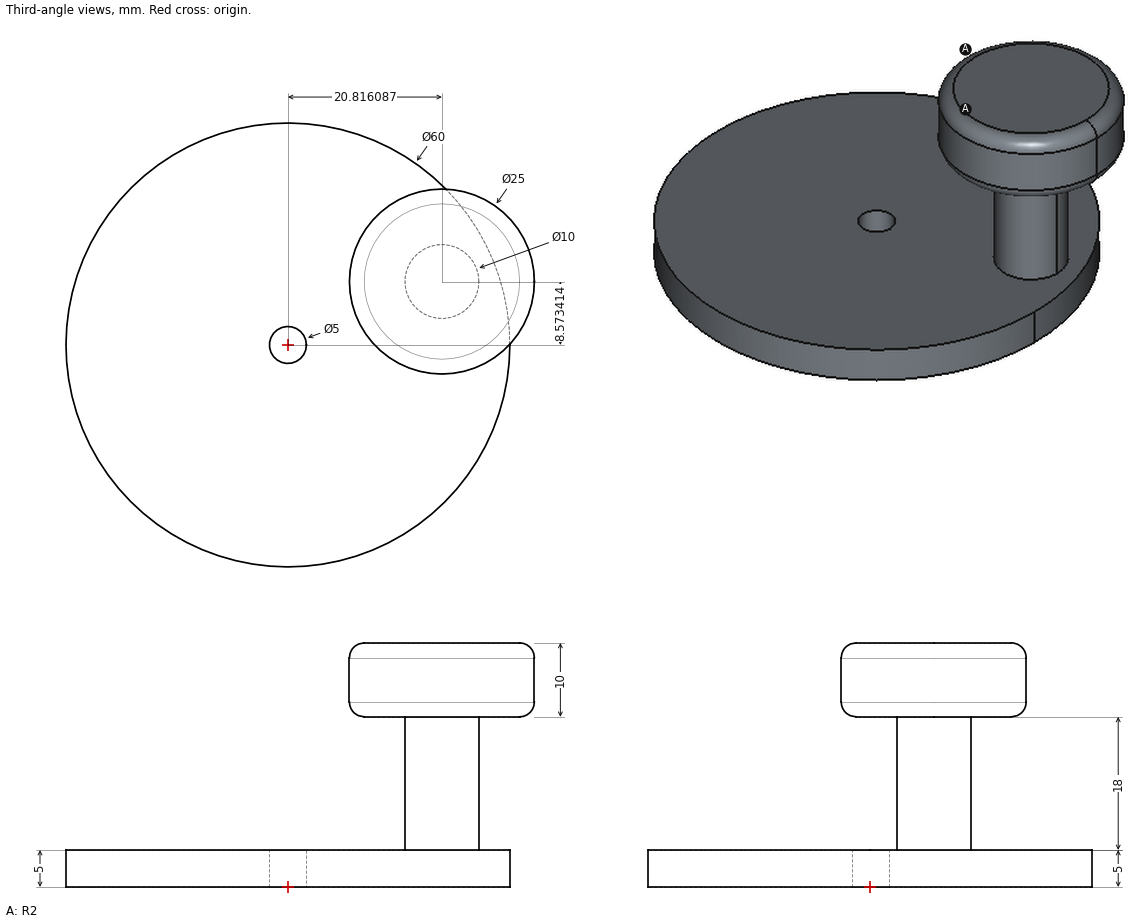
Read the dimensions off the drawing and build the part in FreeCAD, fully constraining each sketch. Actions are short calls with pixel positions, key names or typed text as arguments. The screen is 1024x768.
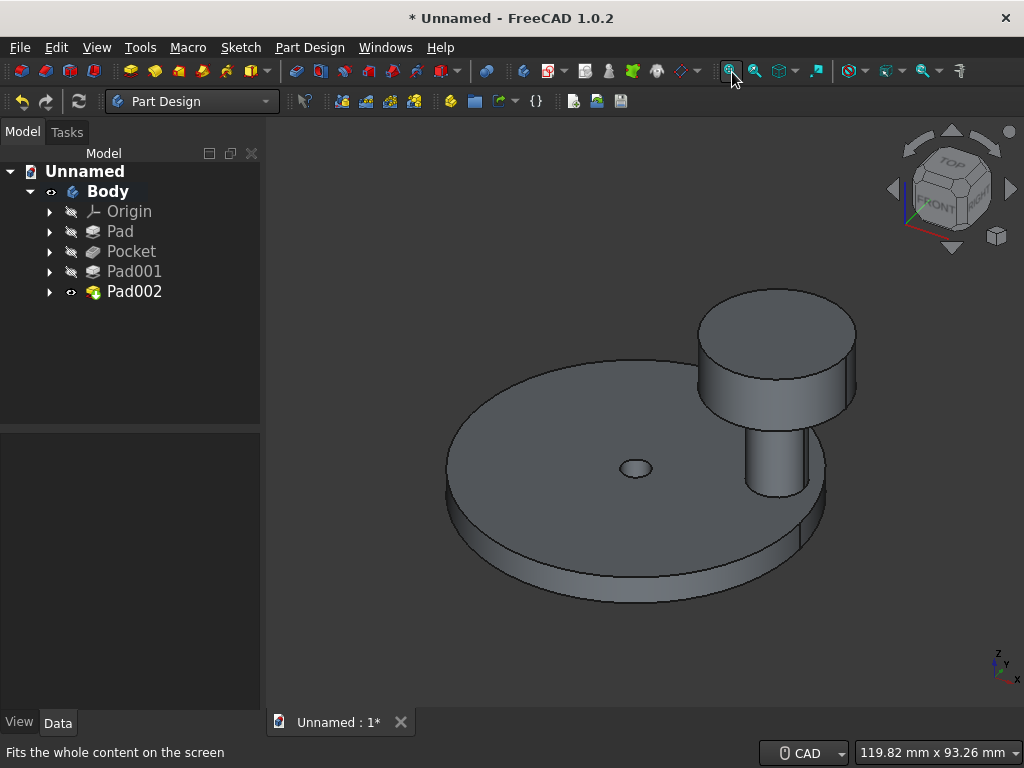
click(698, 338)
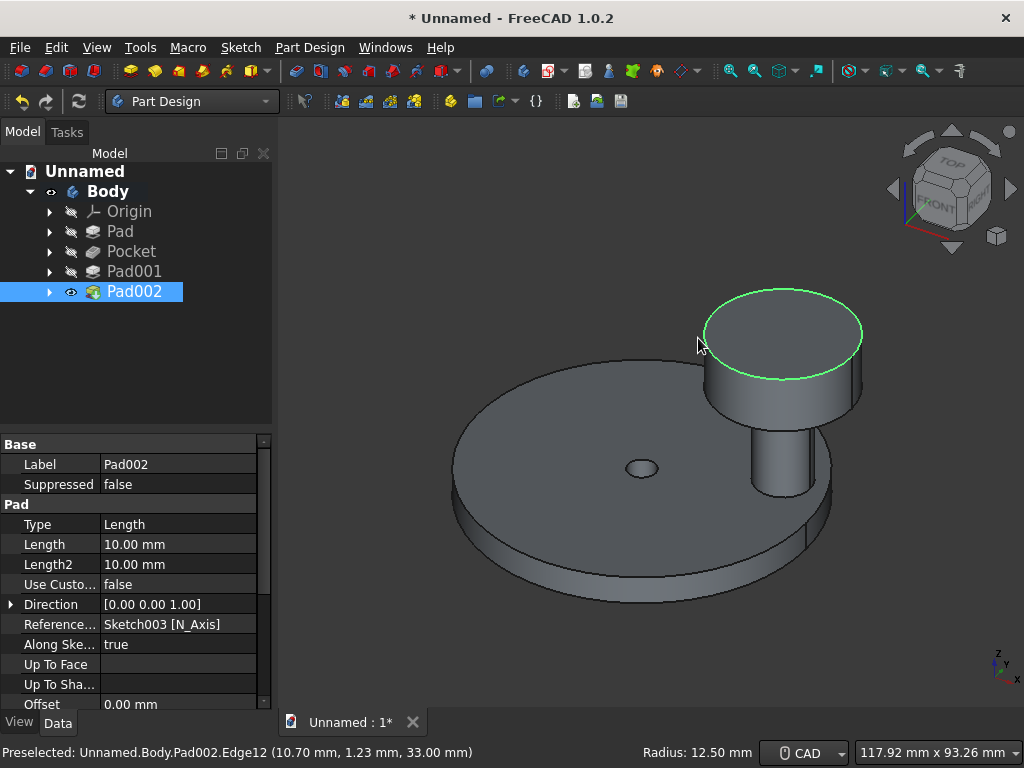
key(0)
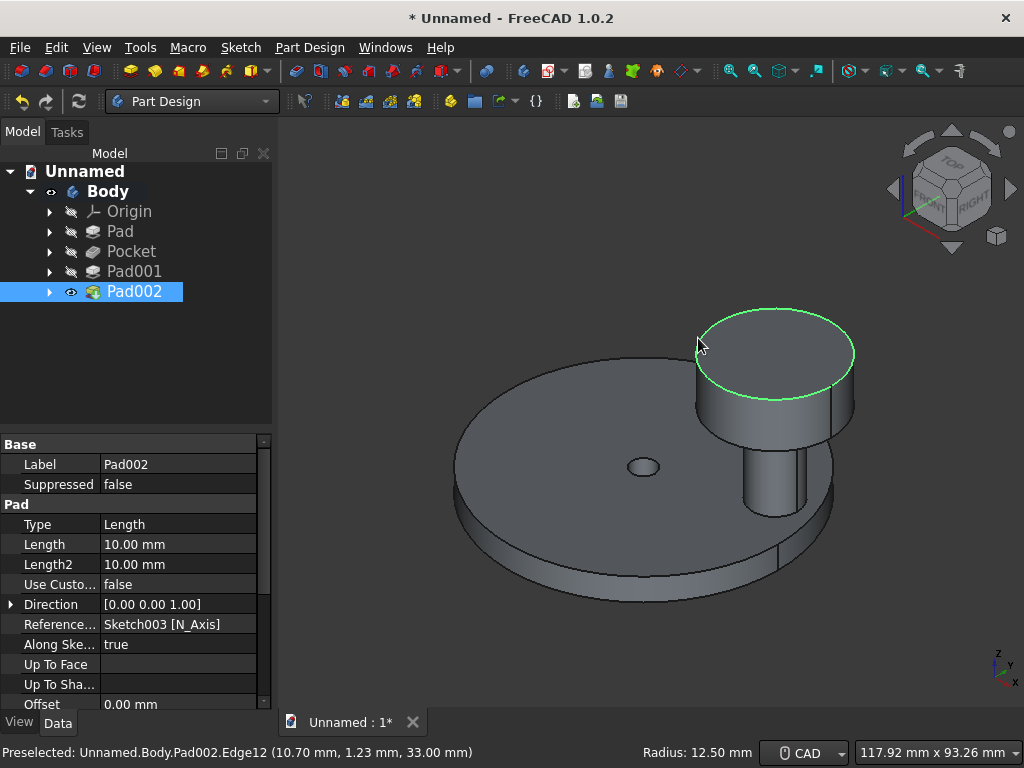
key(2)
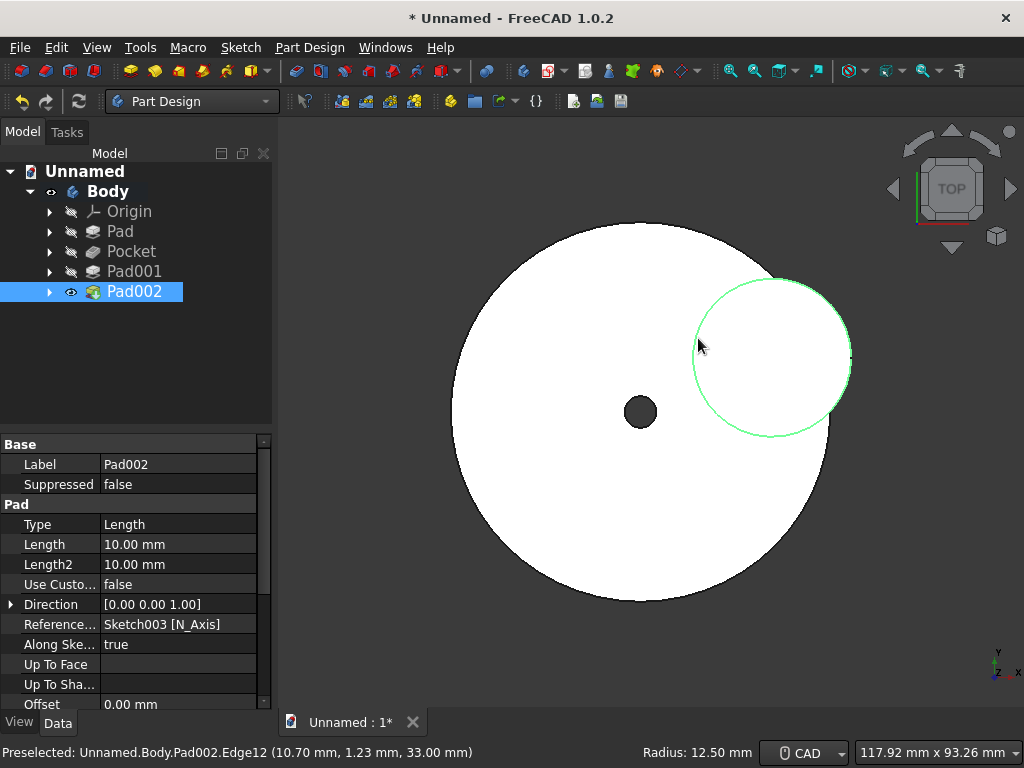
key(1)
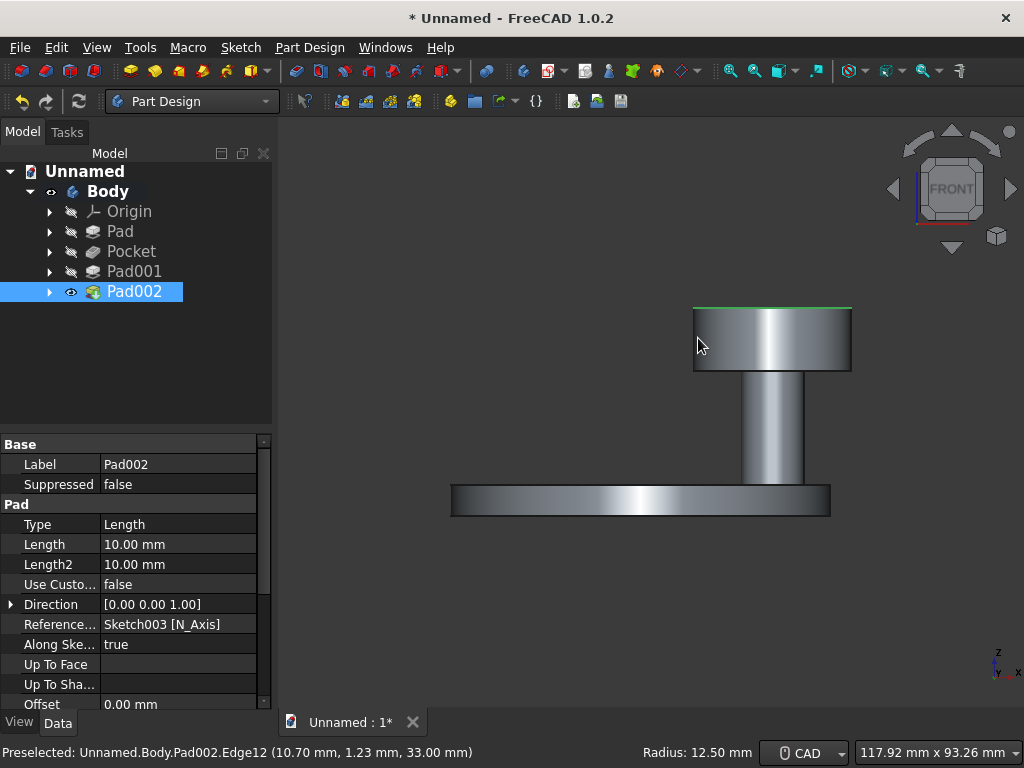
click(708, 370, ctrl)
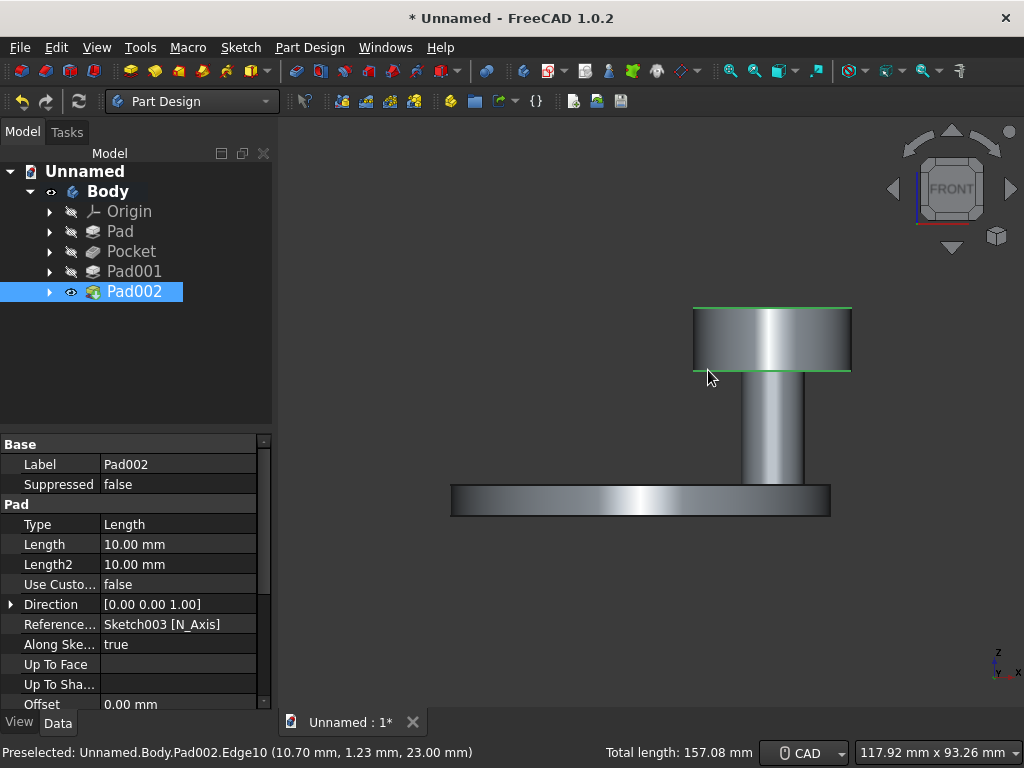
click(22, 72)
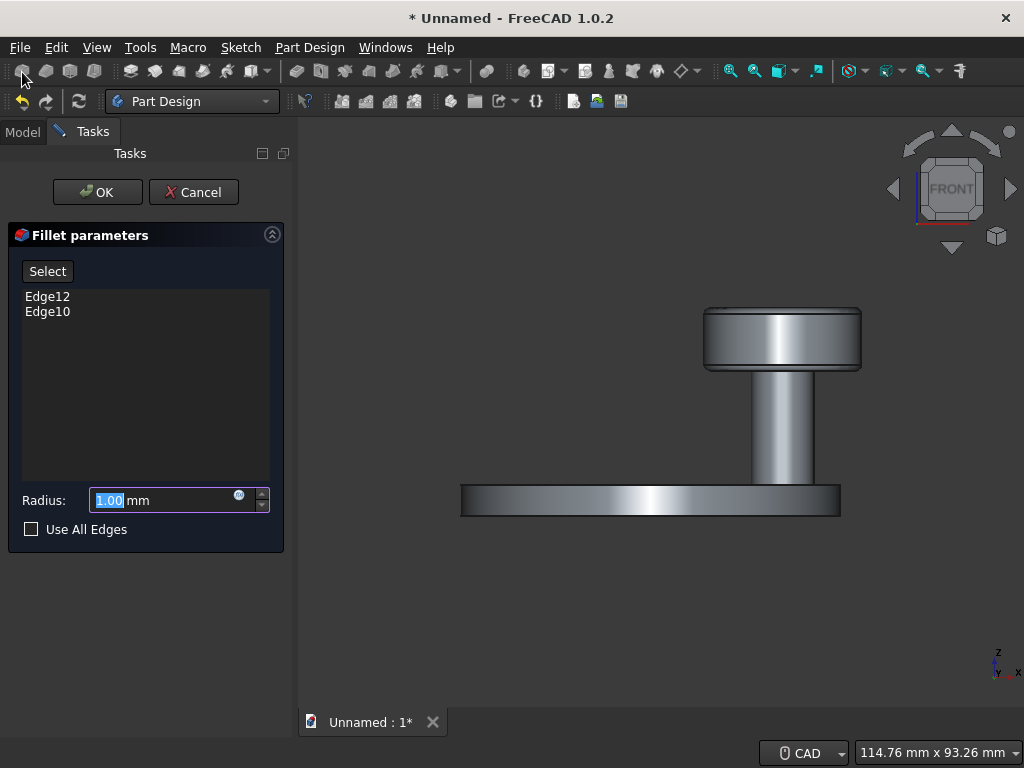
text(2)
key(Tab)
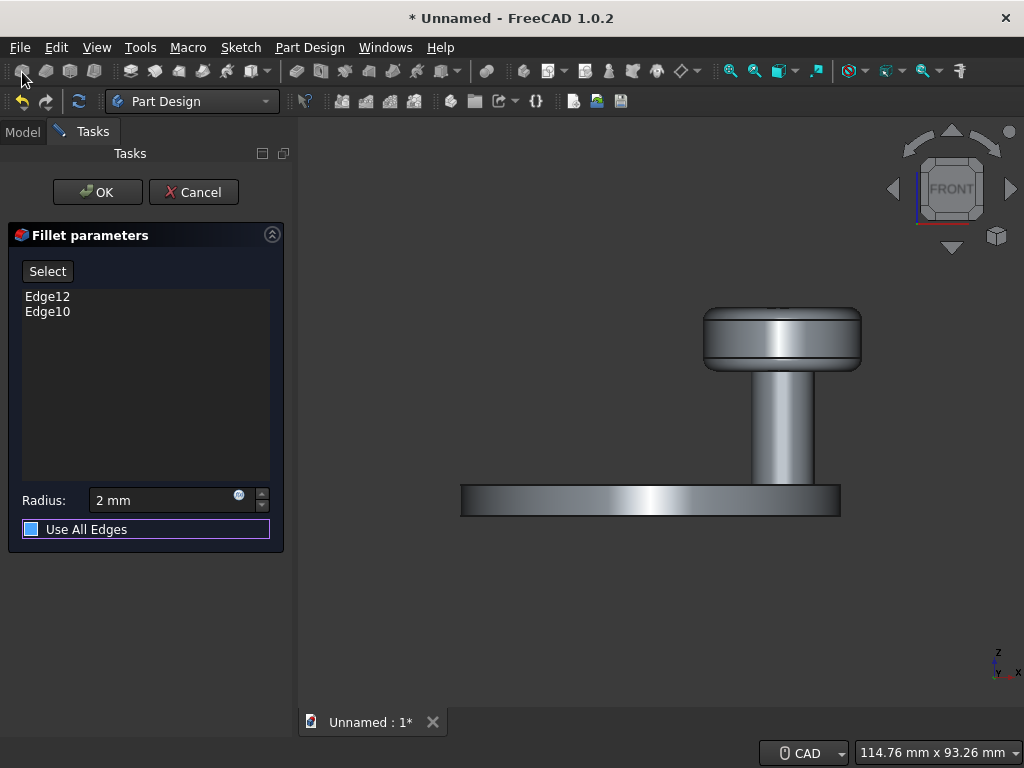
click(98, 192)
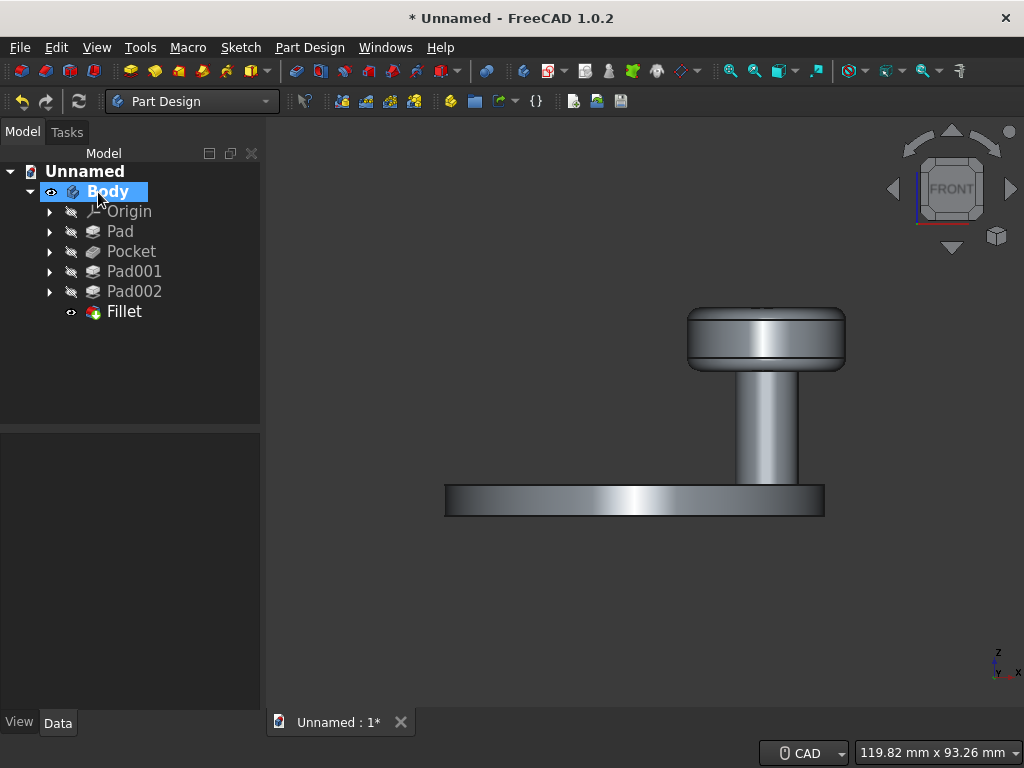
key(0)